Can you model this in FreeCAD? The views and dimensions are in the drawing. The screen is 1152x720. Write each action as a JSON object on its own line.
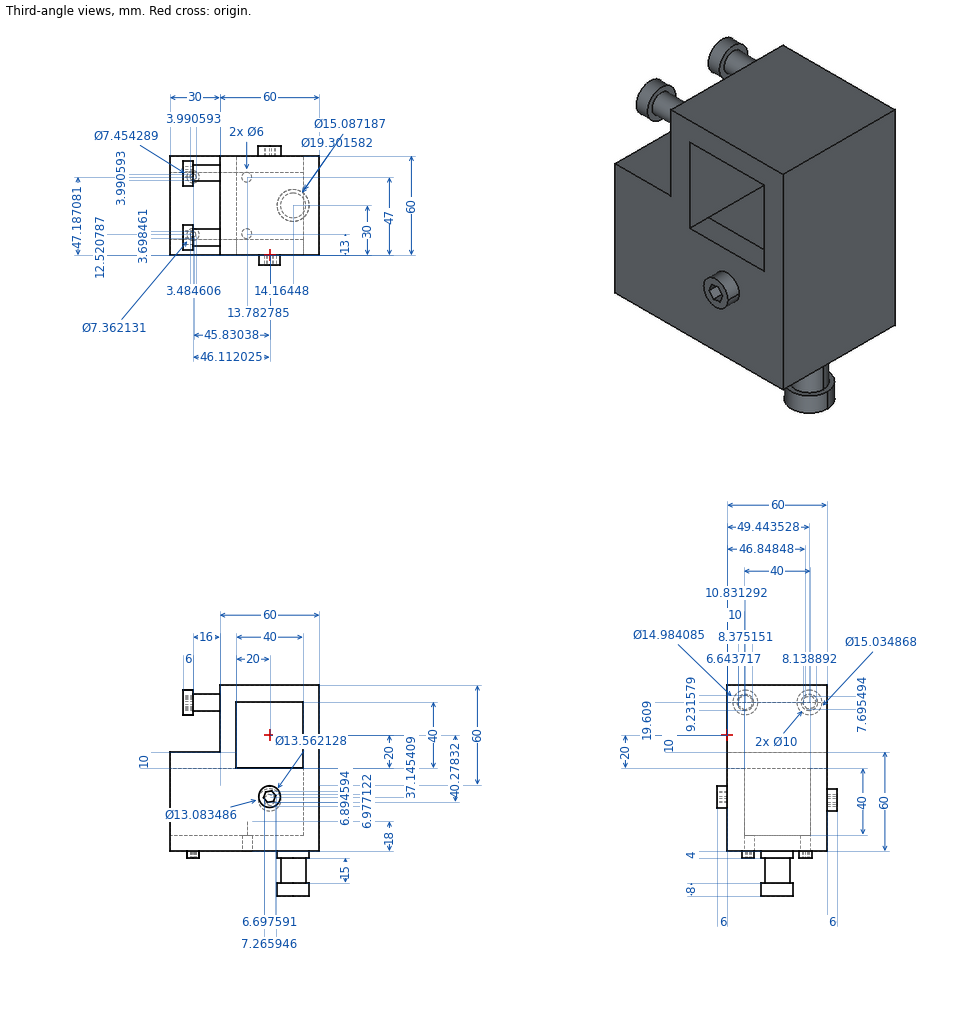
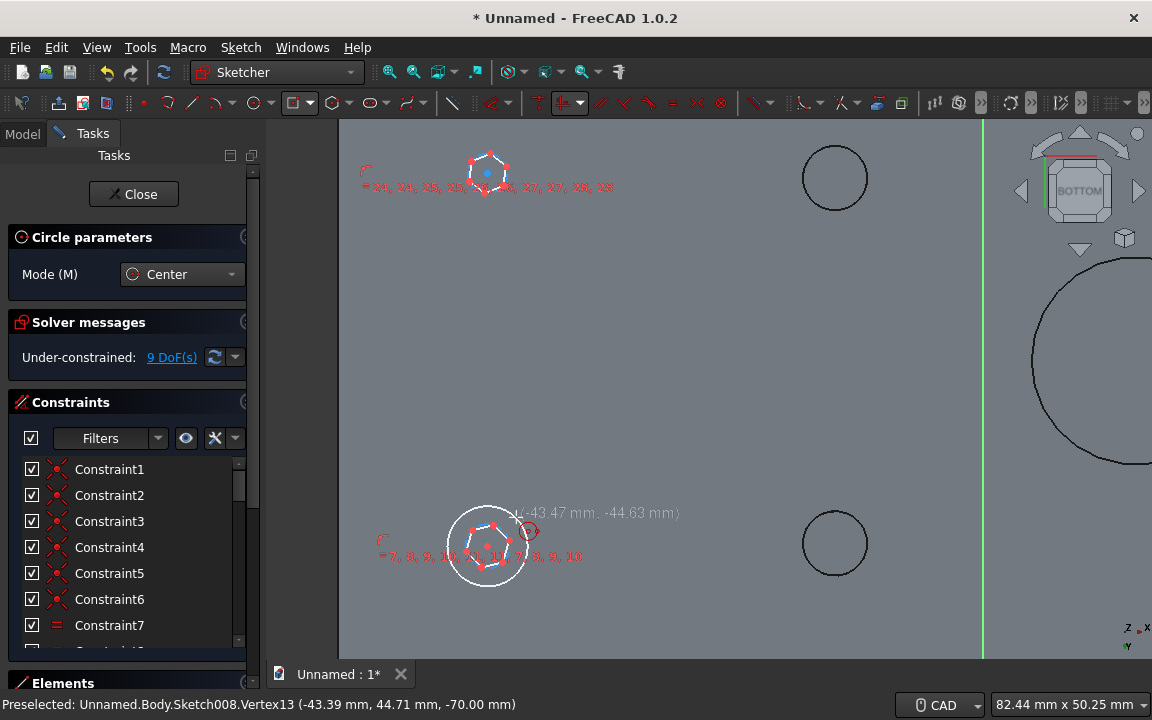
{"action": "left_click", "coordinate": [488, 174]}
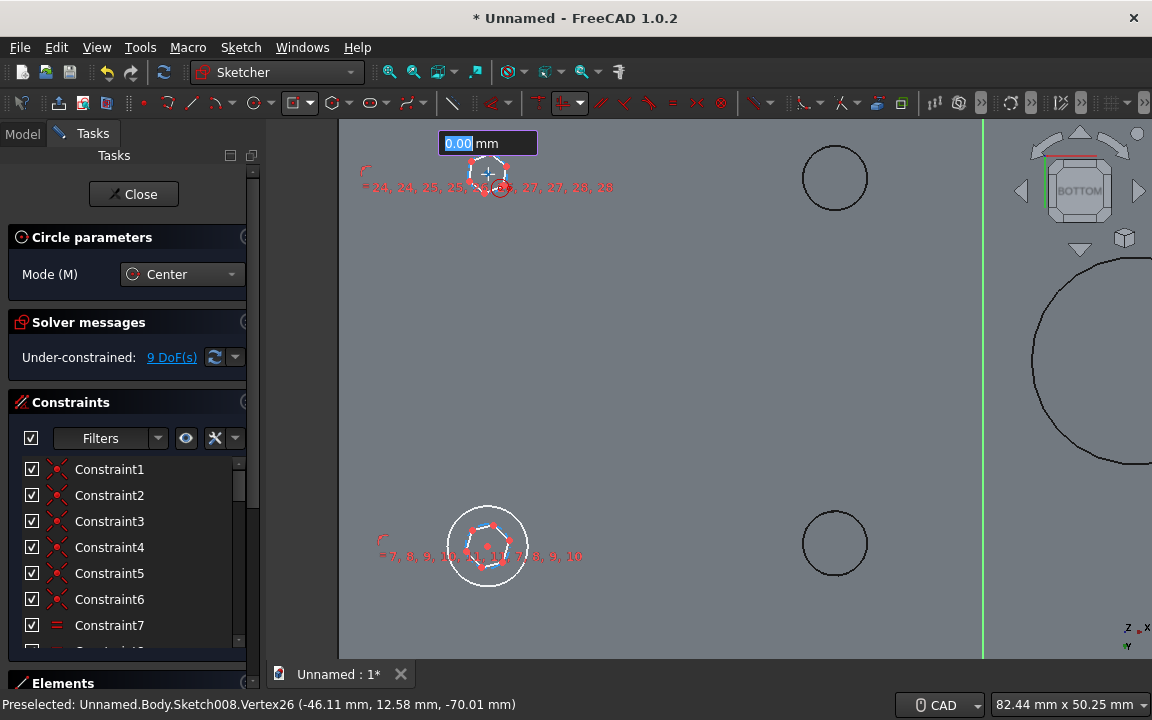
{"action": "scroll", "coordinate": [488, 546], "scroll_direction": "down", "scroll_amount": 2}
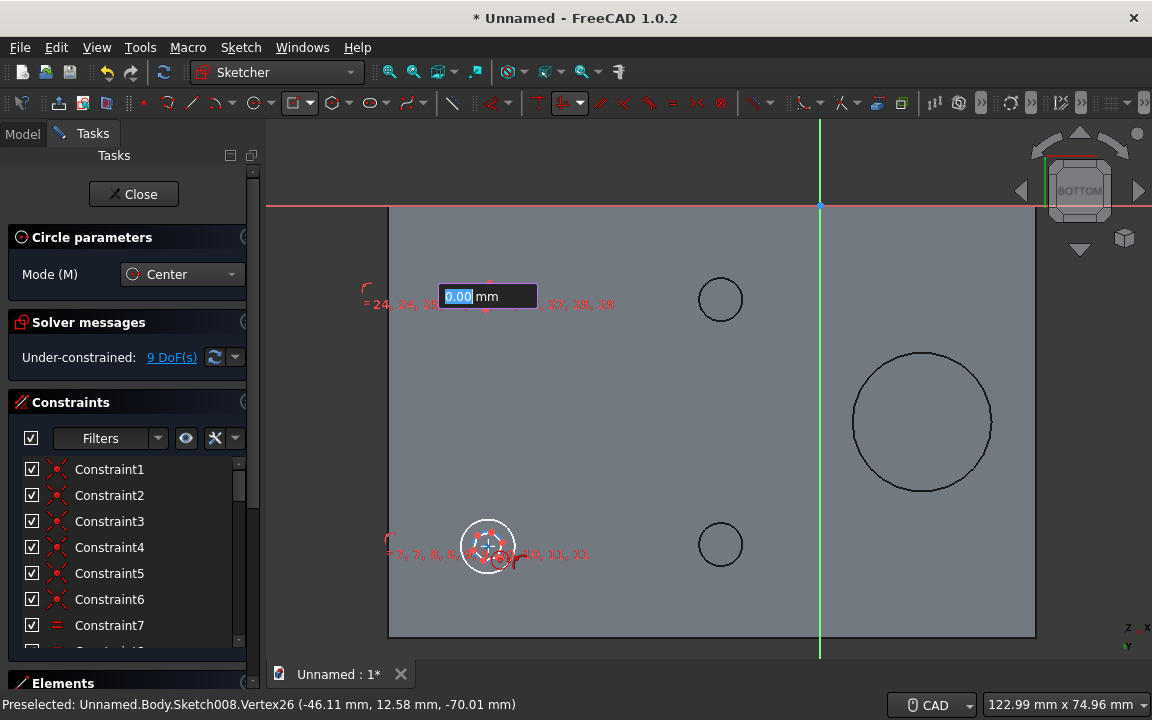
{"action": "left_click", "coordinate": [507, 277]}
{"action": "key", "text": "Escape"}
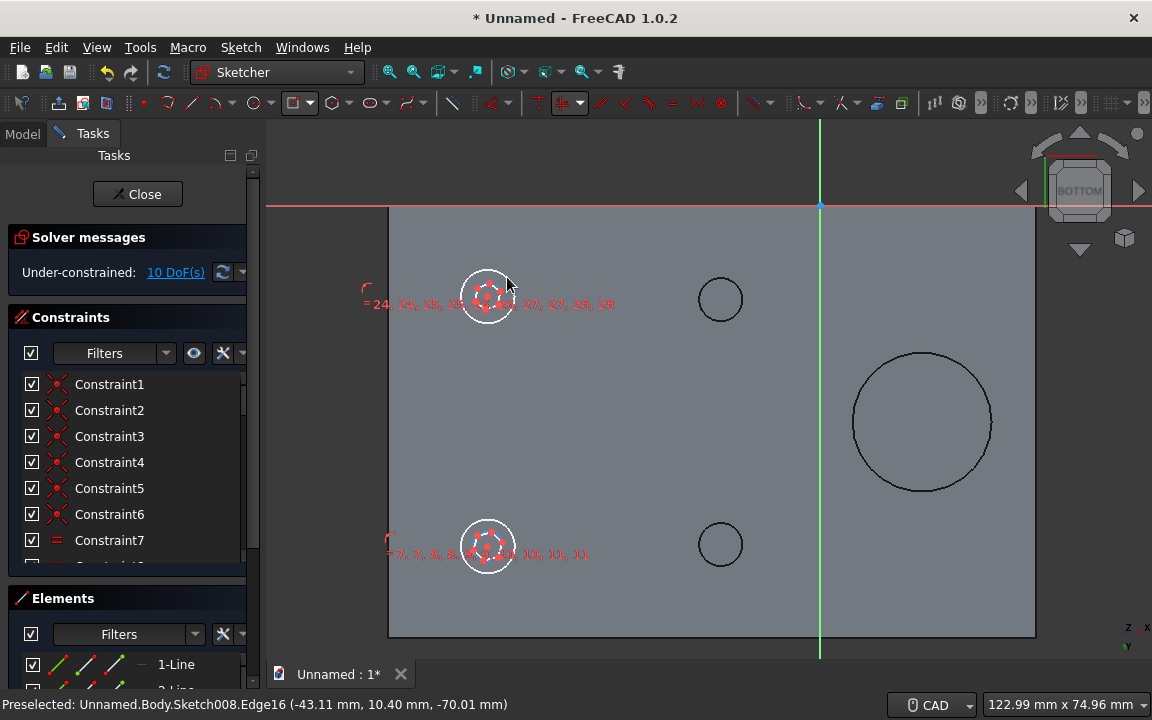
{"action": "left_click", "coordinate": [492, 104]}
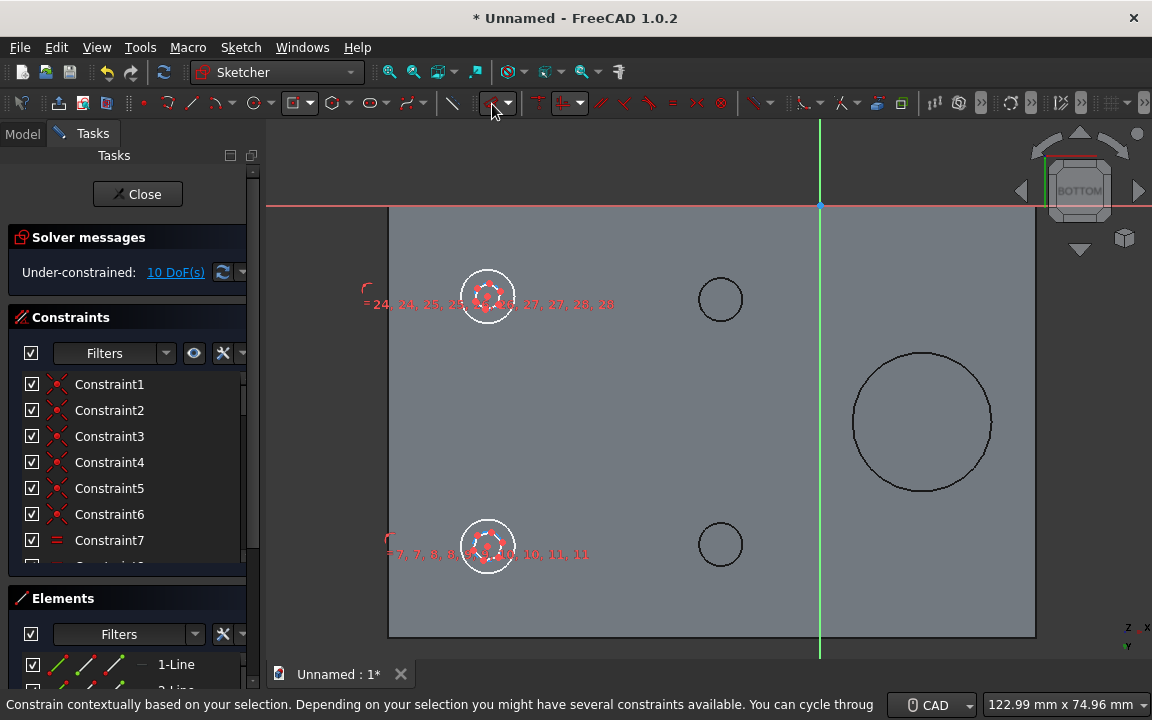
{"action": "left_click", "coordinate": [507, 527]}
{"action": "left_click", "coordinate": [529, 504]}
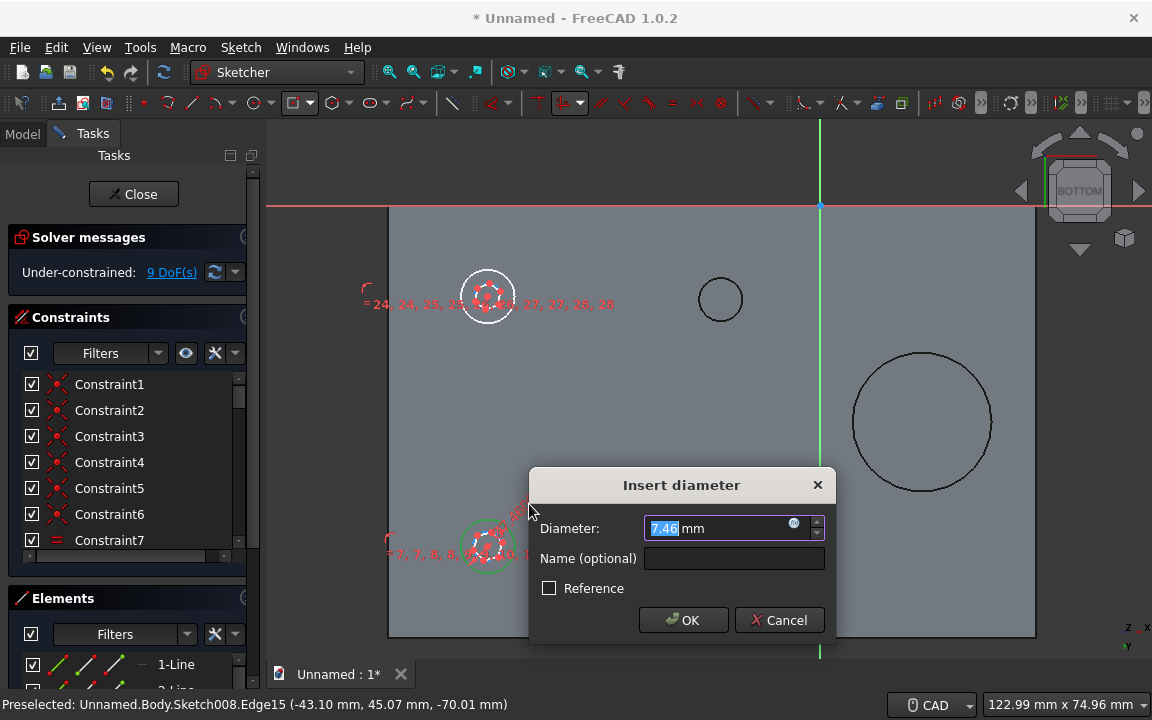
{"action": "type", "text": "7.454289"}
{"action": "key", "text": "Return"}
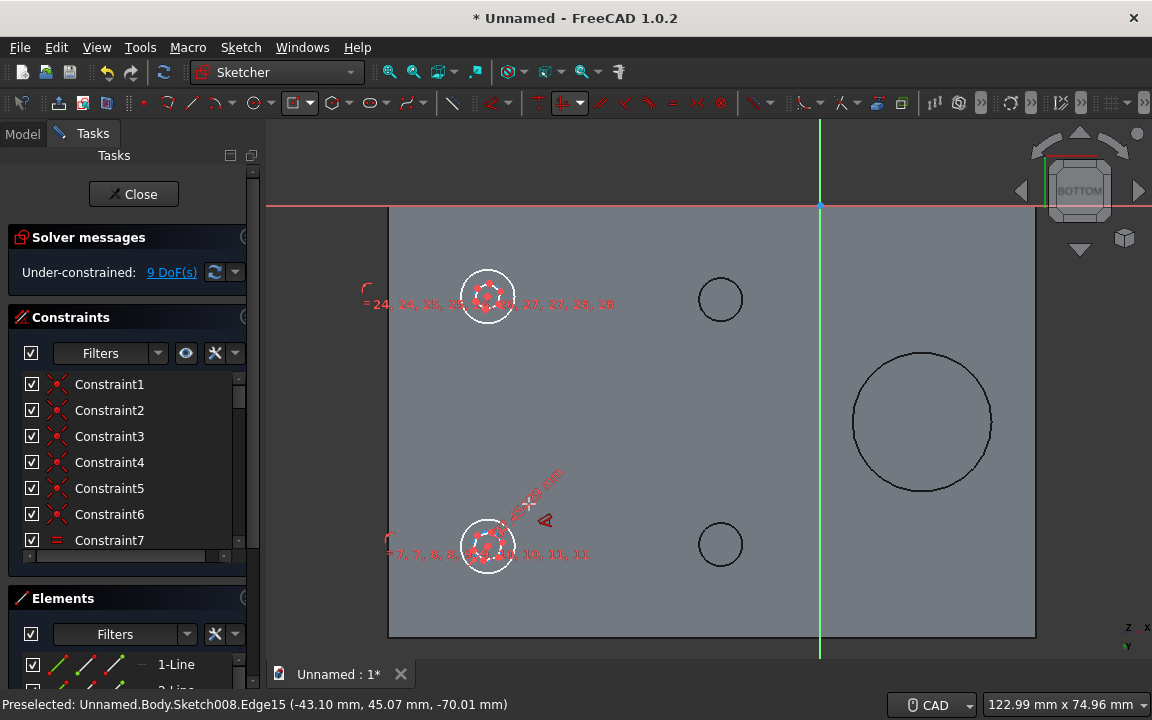
{"action": "left_click", "coordinate": [507, 278]}
{"action": "left_click", "coordinate": [530, 256]}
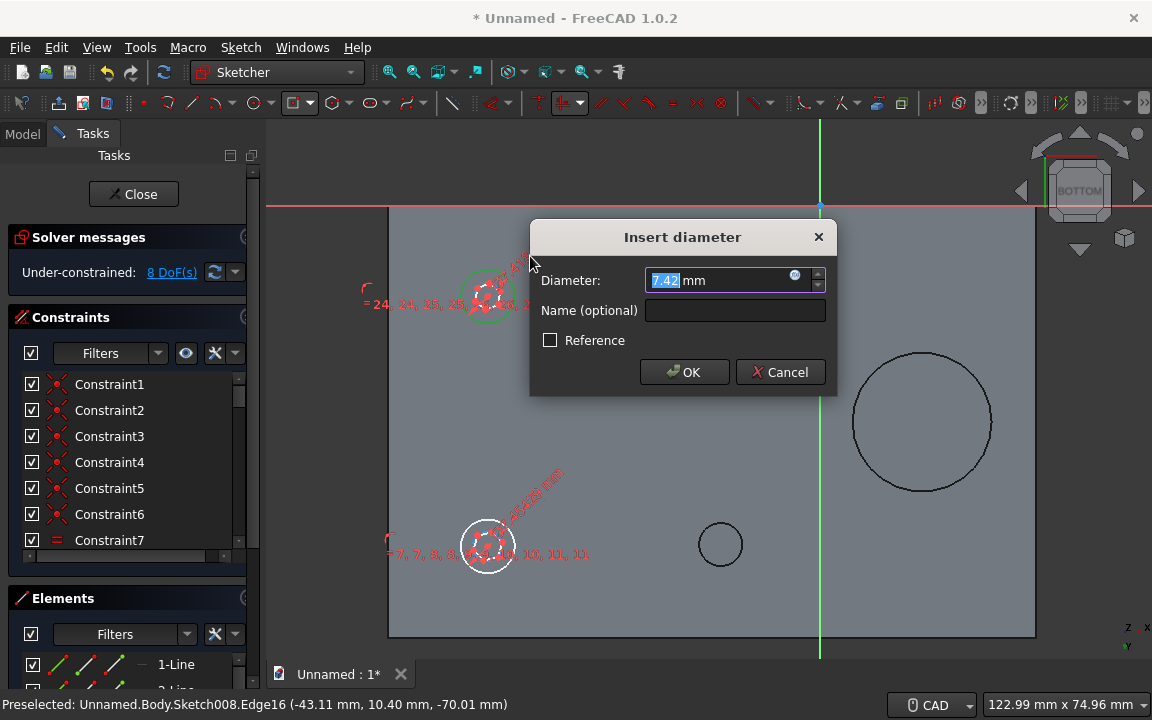
{"action": "type", "text": "7.362131"}
{"action": "key", "text": "Return"}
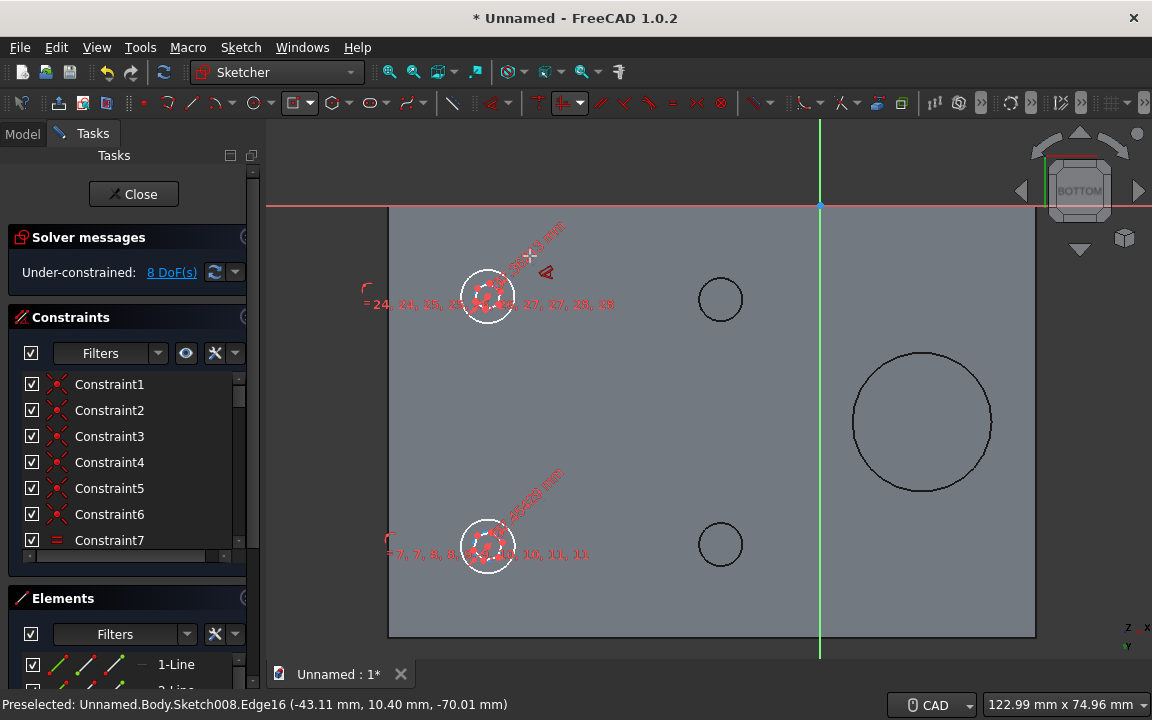
{"action": "scroll", "coordinate": [473, 550], "scroll_direction": "up", "scroll_amount": 2}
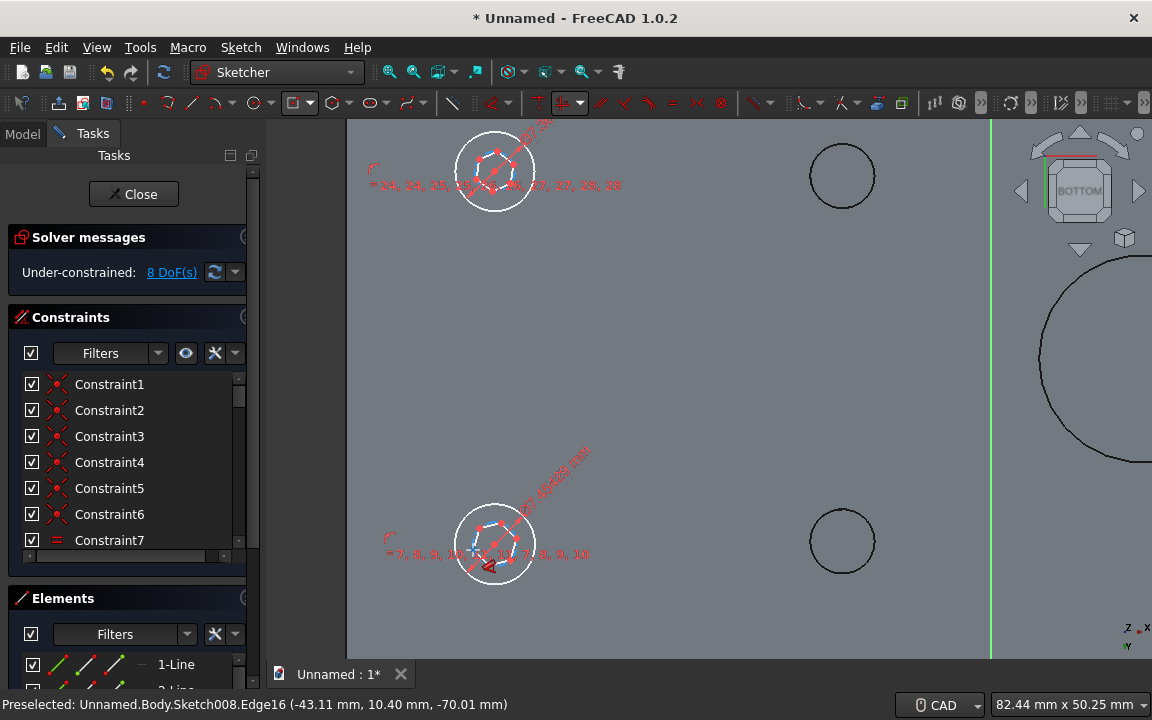
{"action": "left_click", "coordinate": [473, 550]}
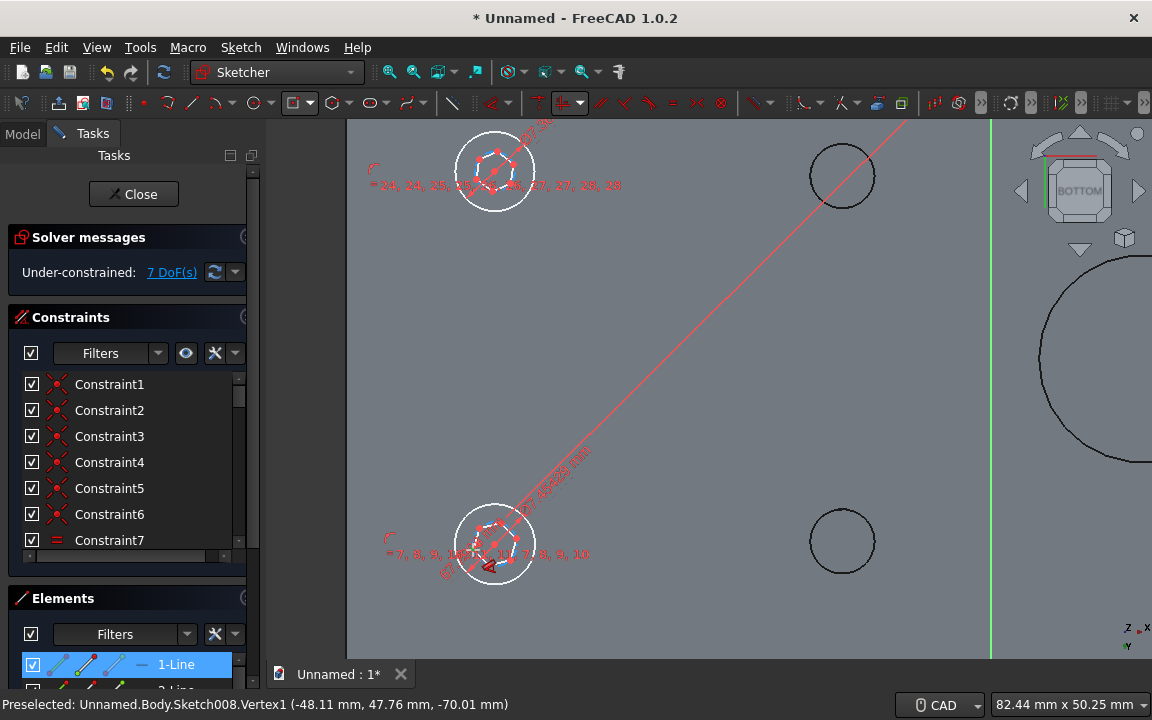
{"action": "left_click", "coordinate": [516, 539]}
{"action": "left_click", "coordinate": [495, 608]}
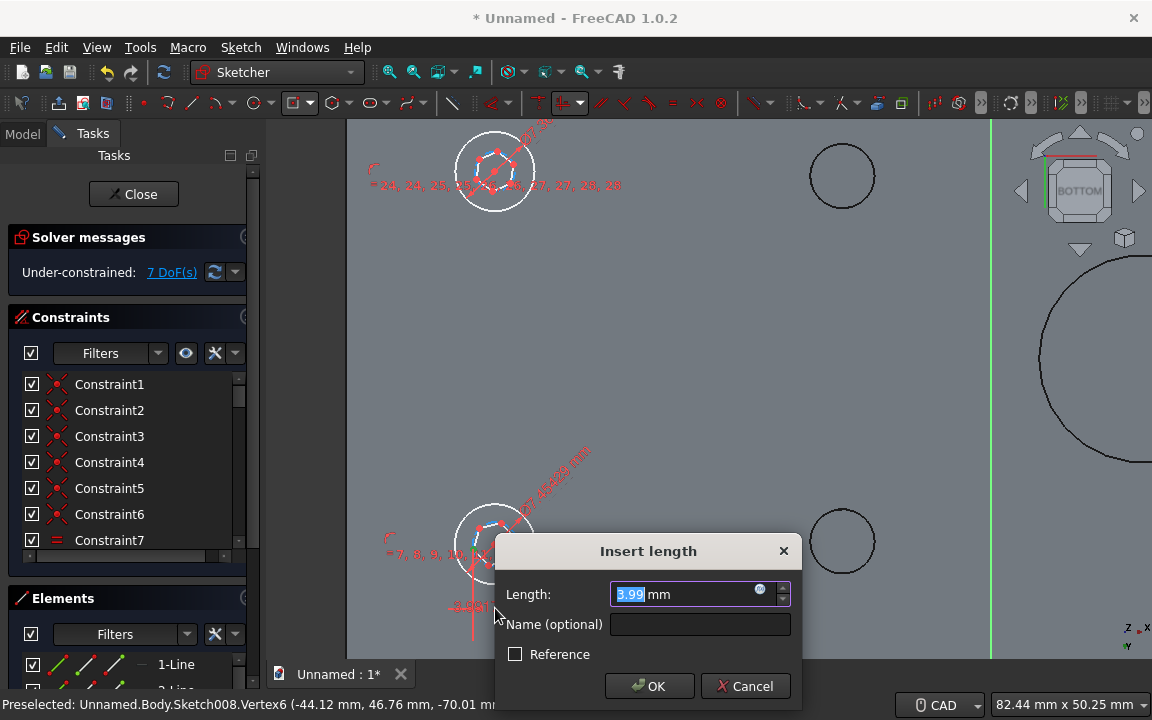
{"action": "type", "text": "3.990593"}
{"action": "key", "text": "Return"}